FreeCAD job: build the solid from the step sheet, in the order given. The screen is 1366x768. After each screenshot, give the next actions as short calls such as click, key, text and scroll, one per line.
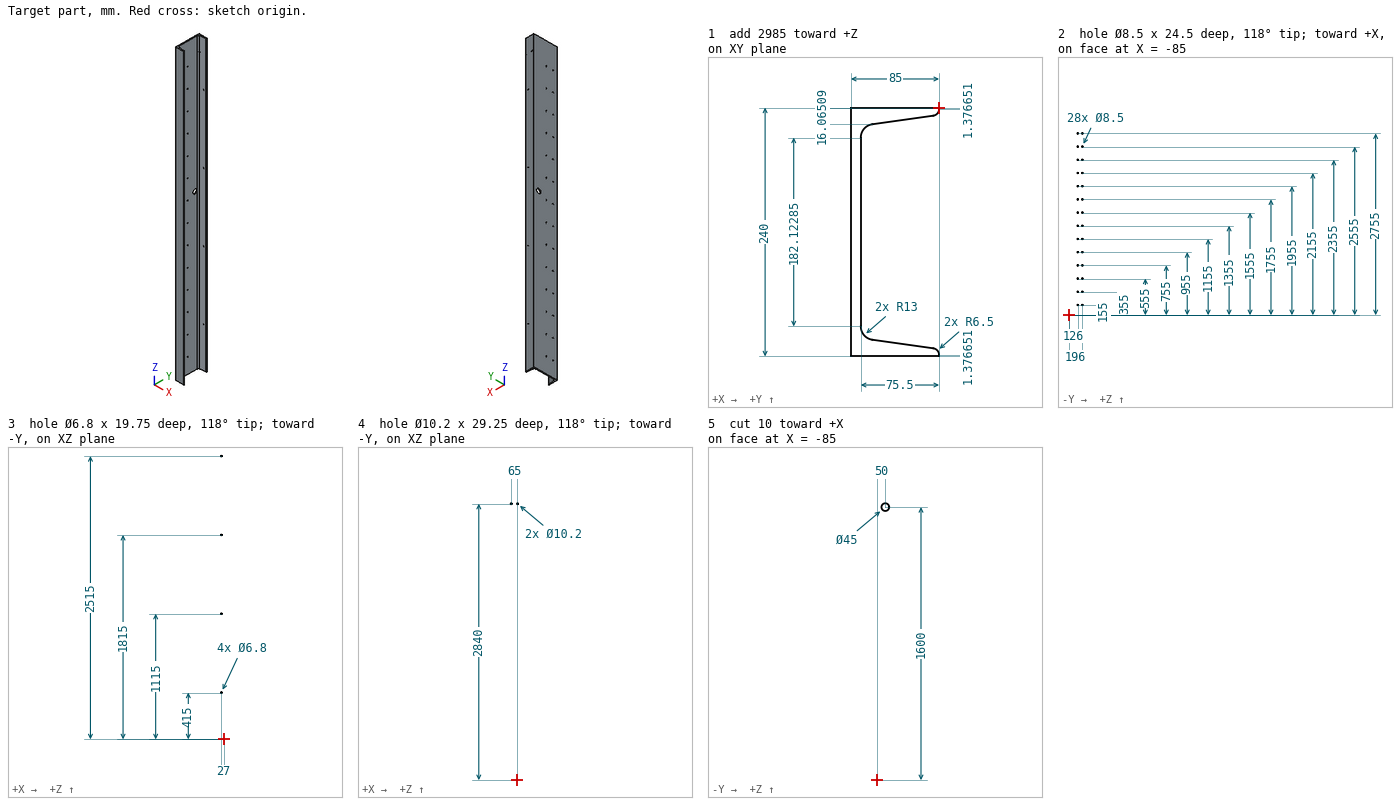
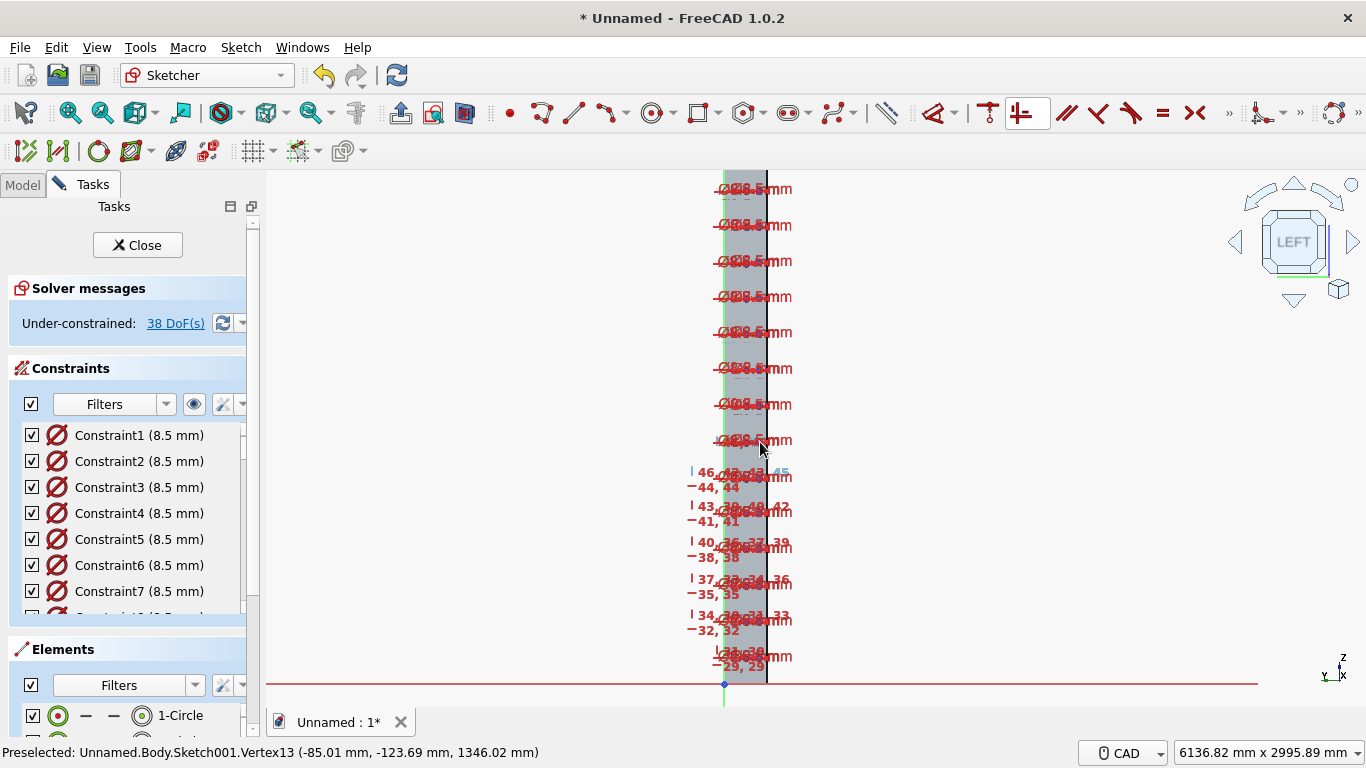
scroll(759, 442, up, 4)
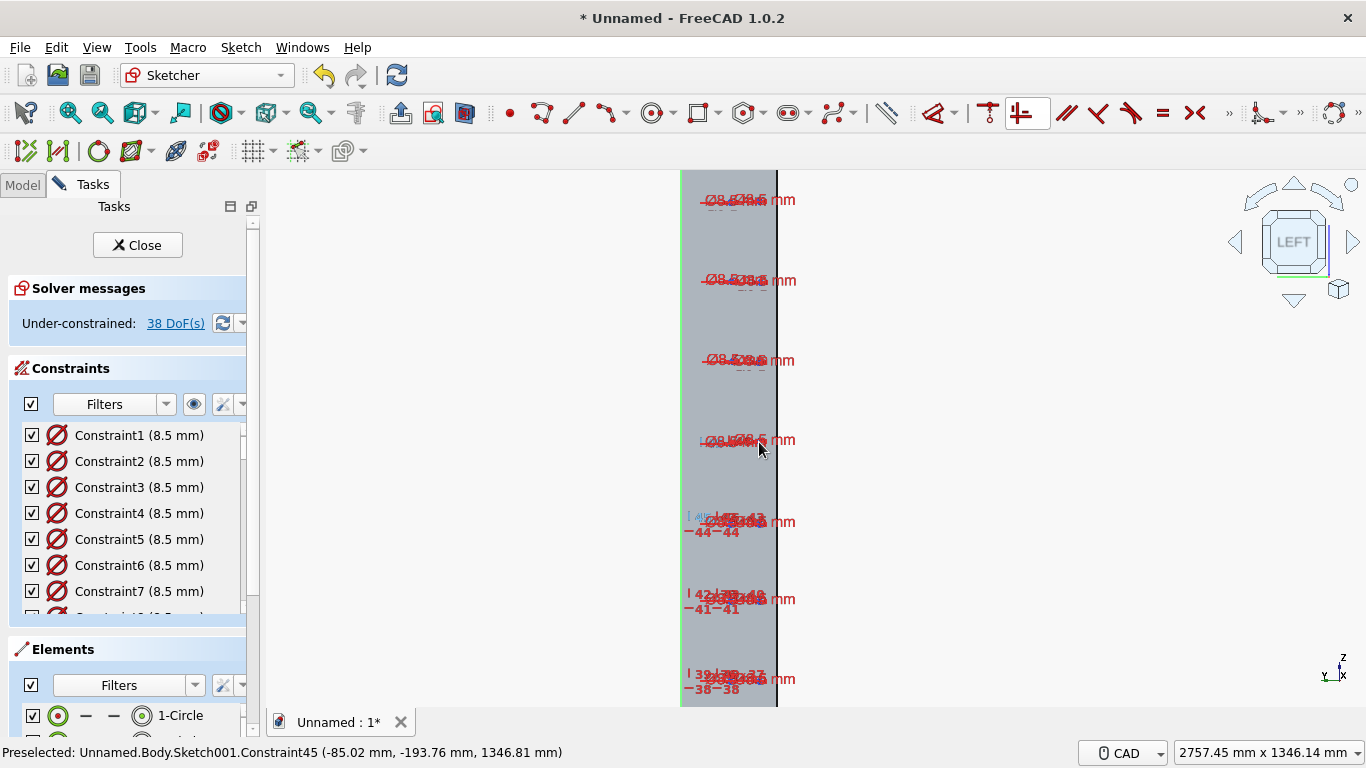
click(759, 442)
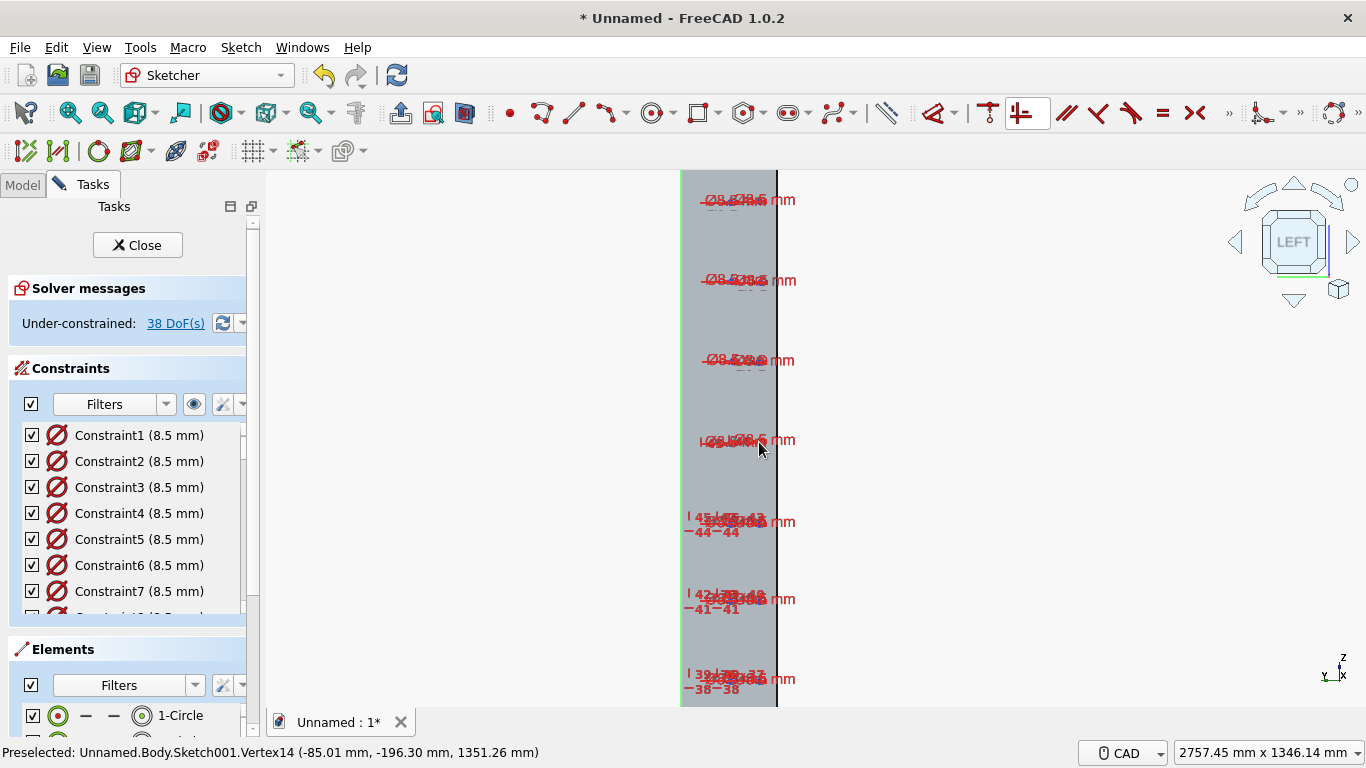
click(1044, 114)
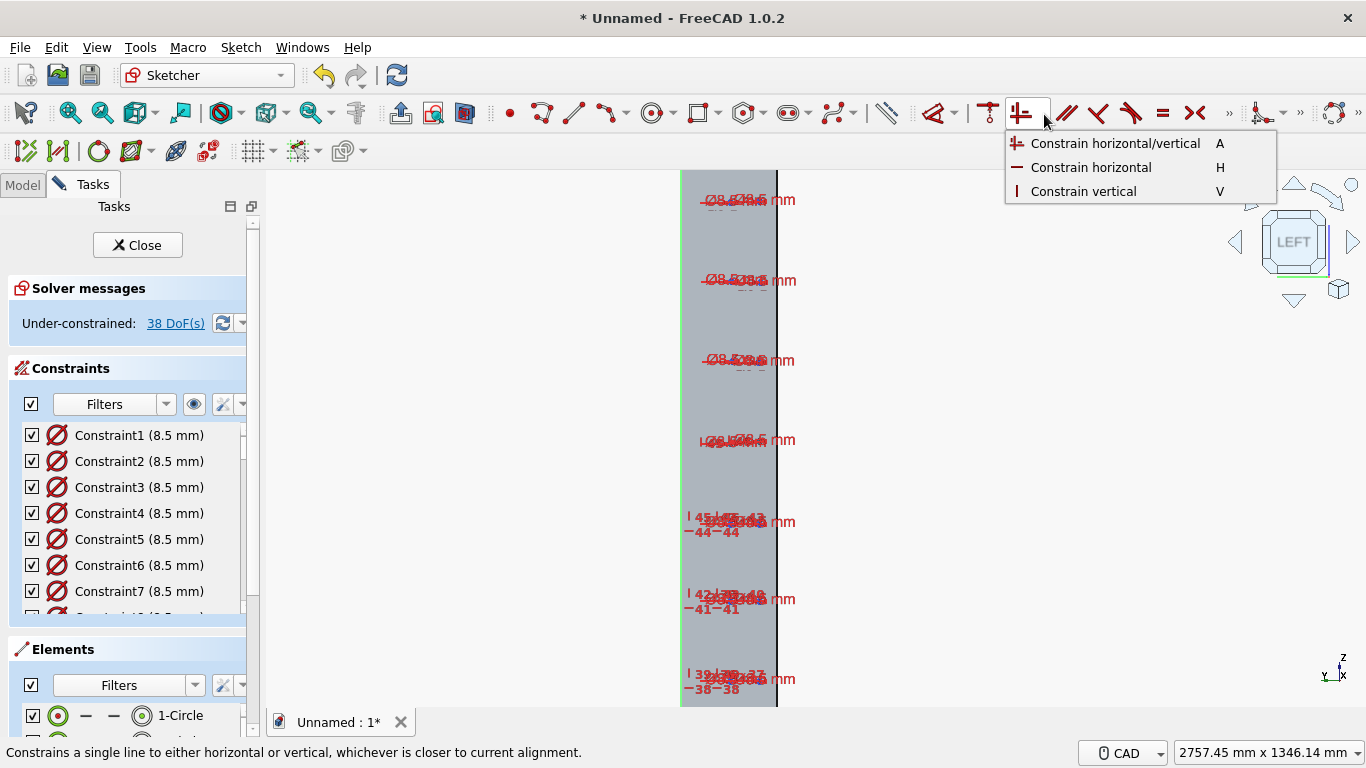
click(1141, 167)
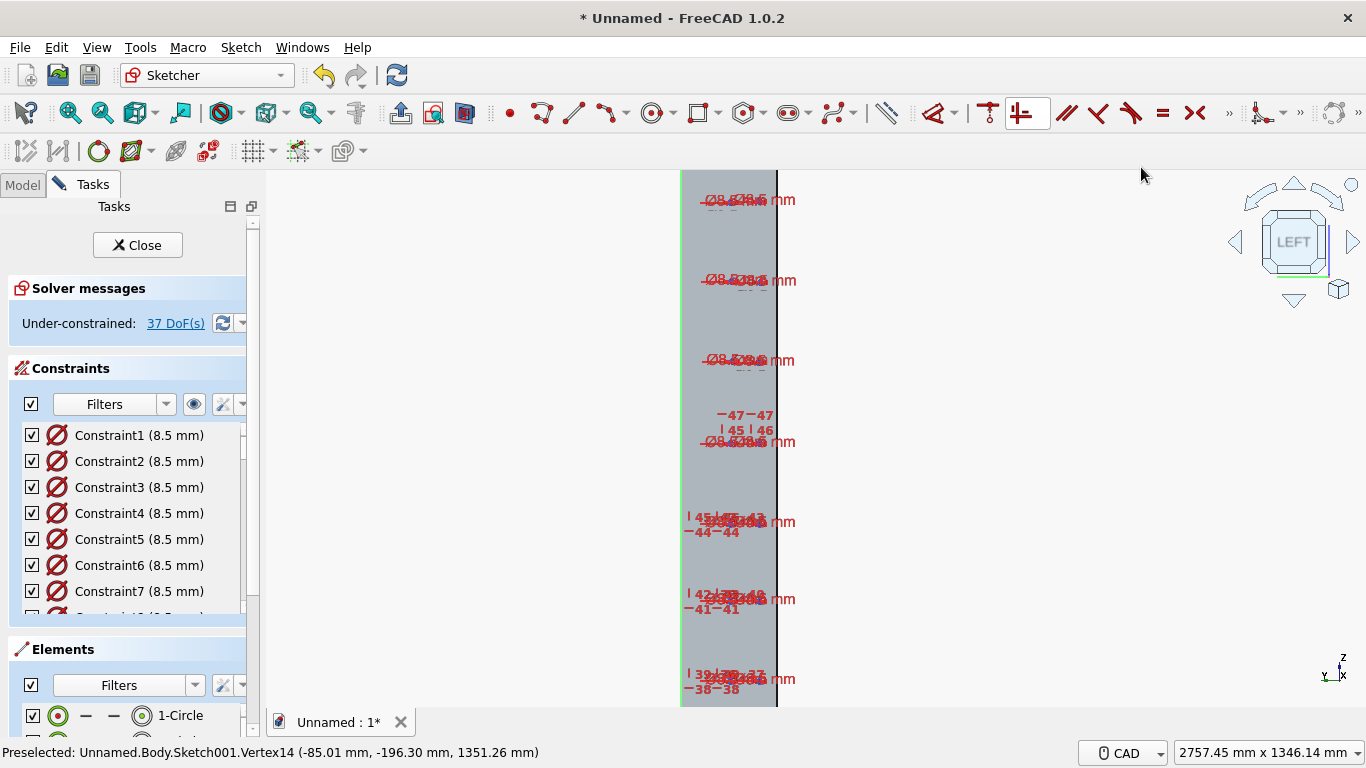
click(759, 444)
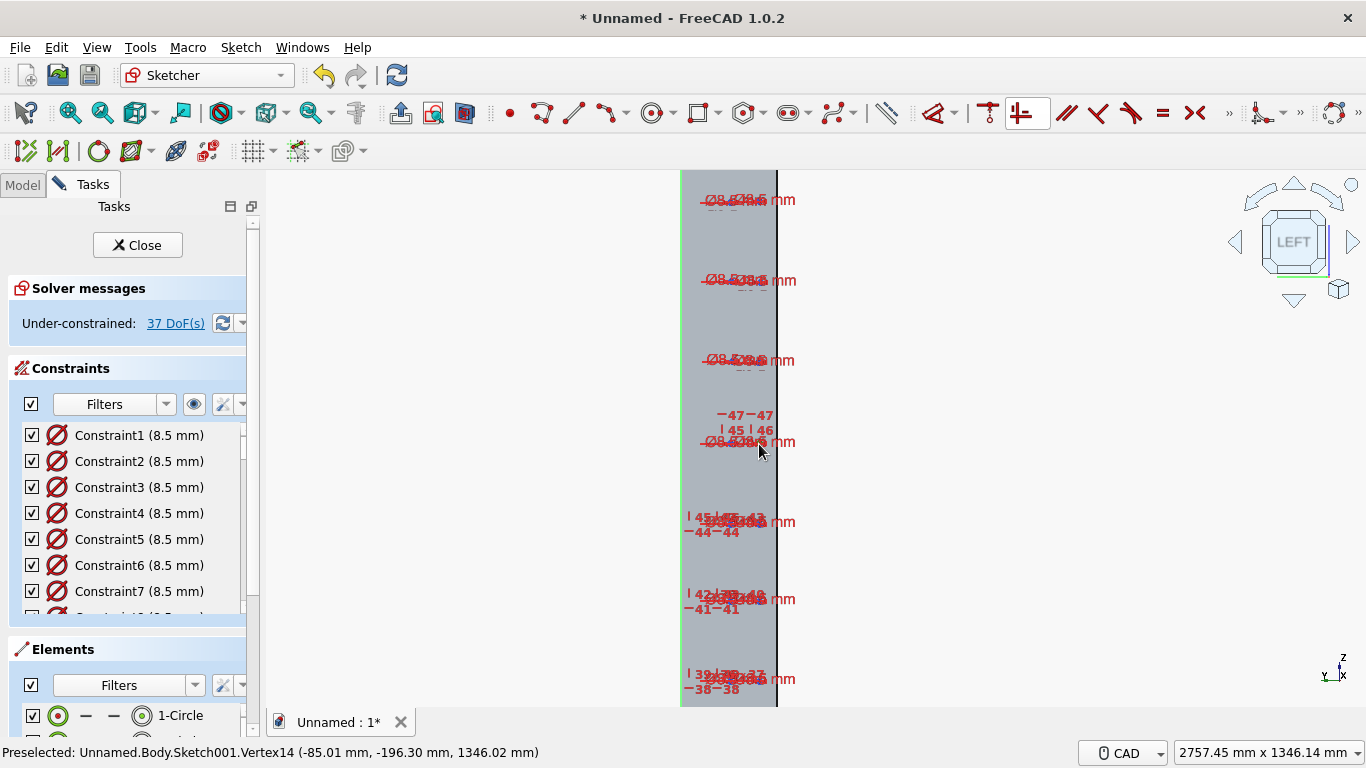
click(759, 363)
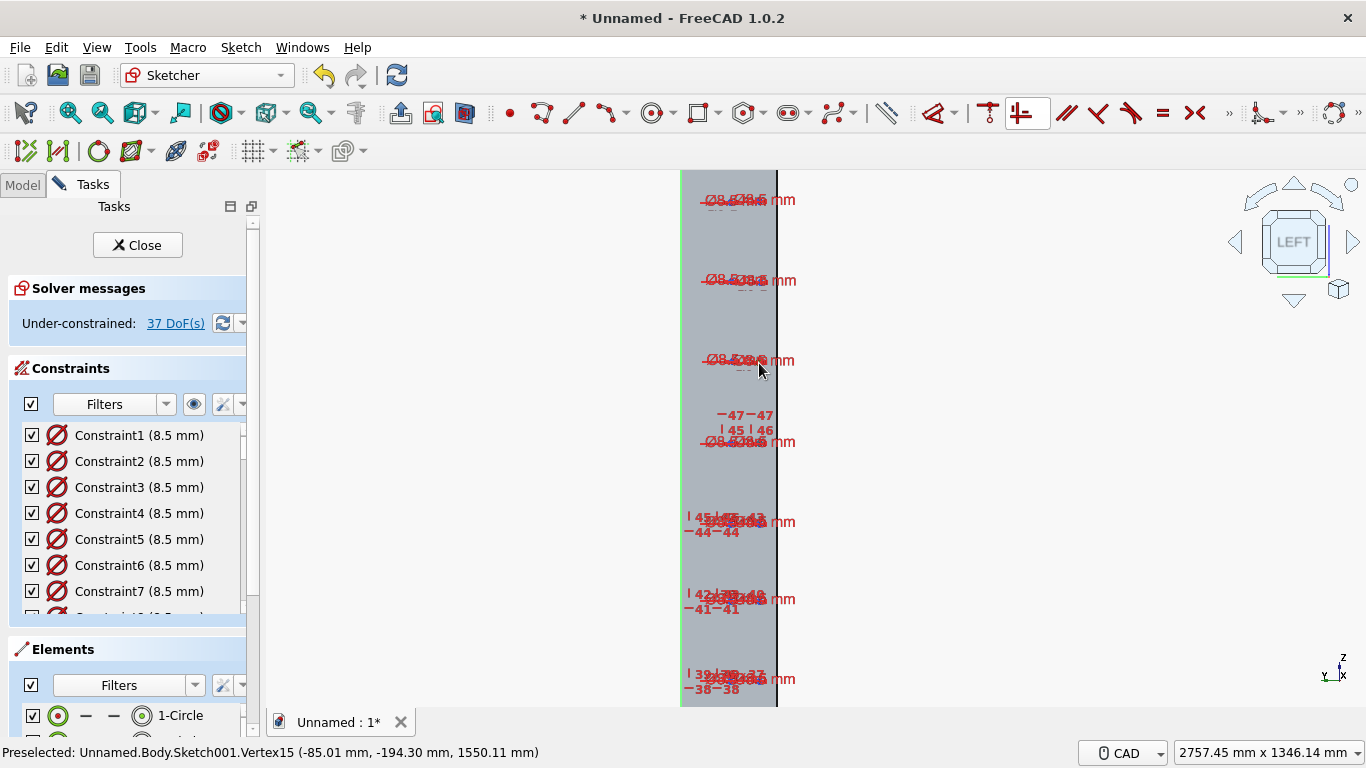
click(1044, 114)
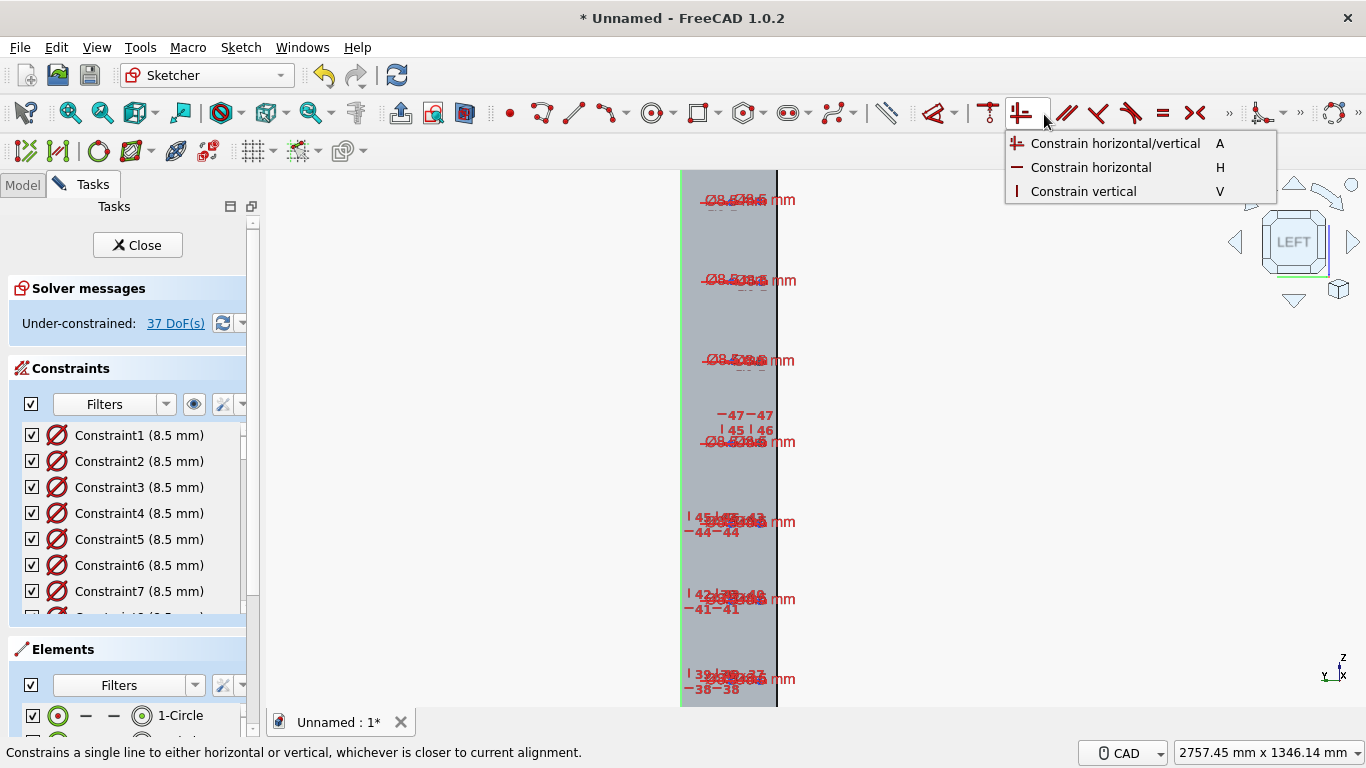
click(1141, 191)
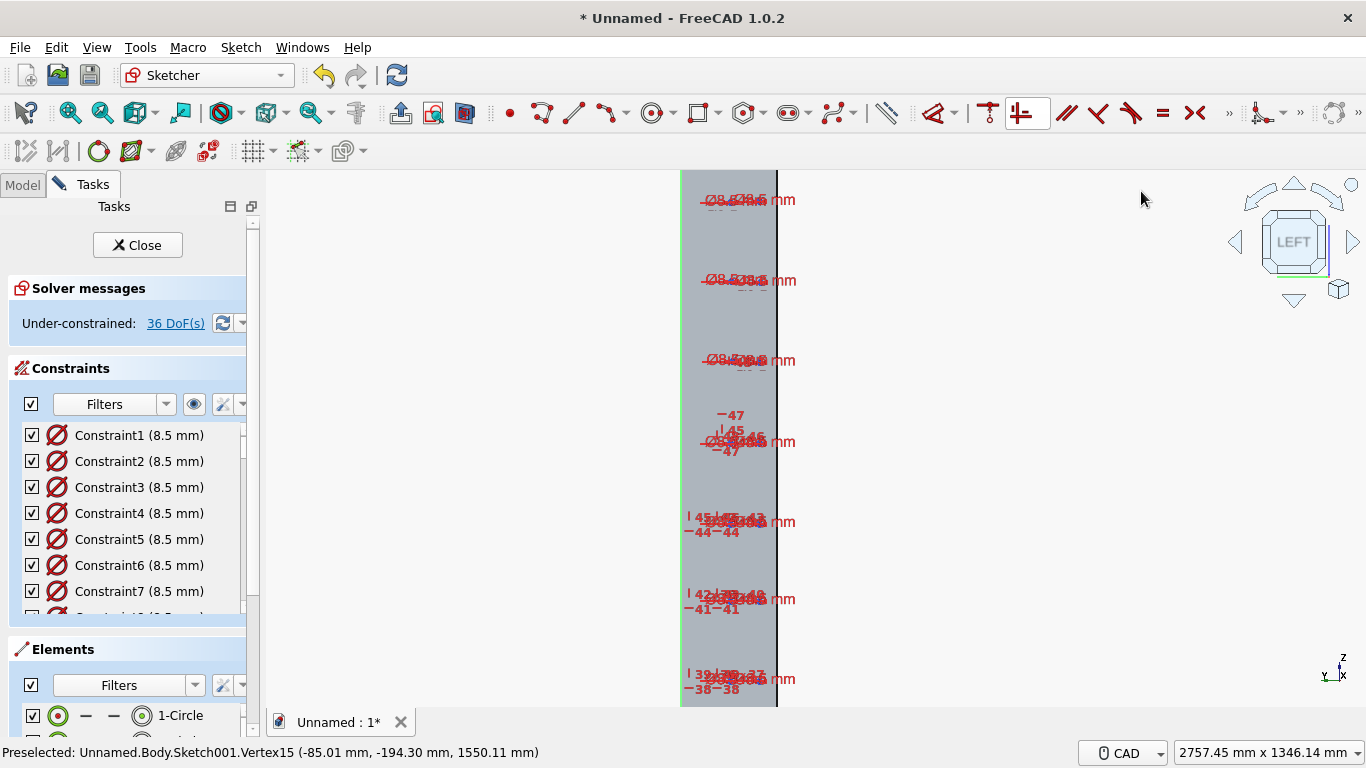
click(730, 444)